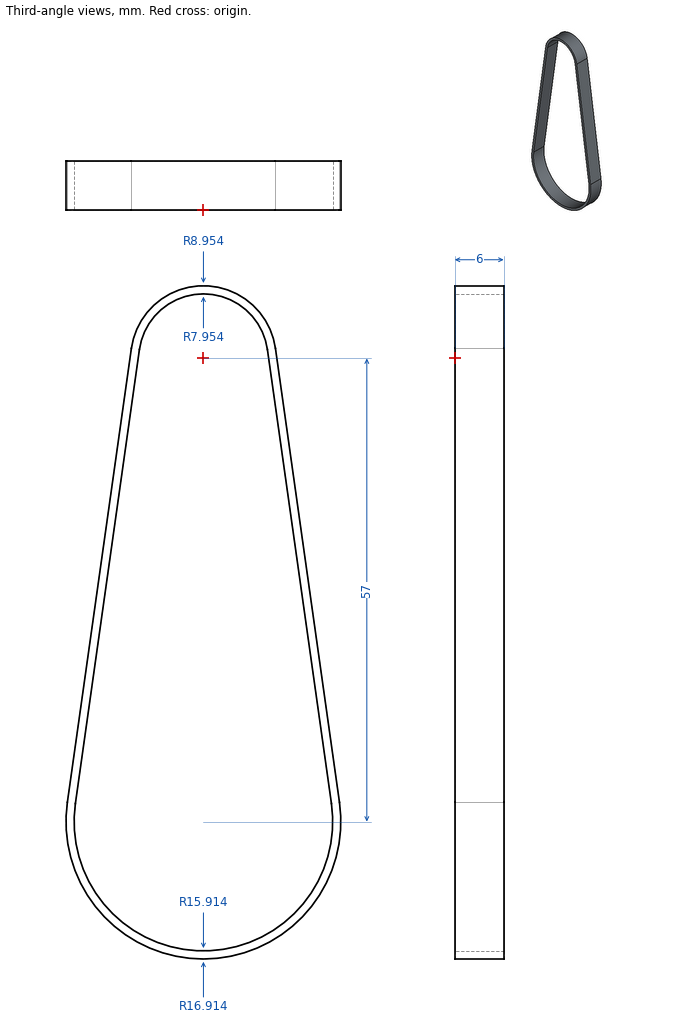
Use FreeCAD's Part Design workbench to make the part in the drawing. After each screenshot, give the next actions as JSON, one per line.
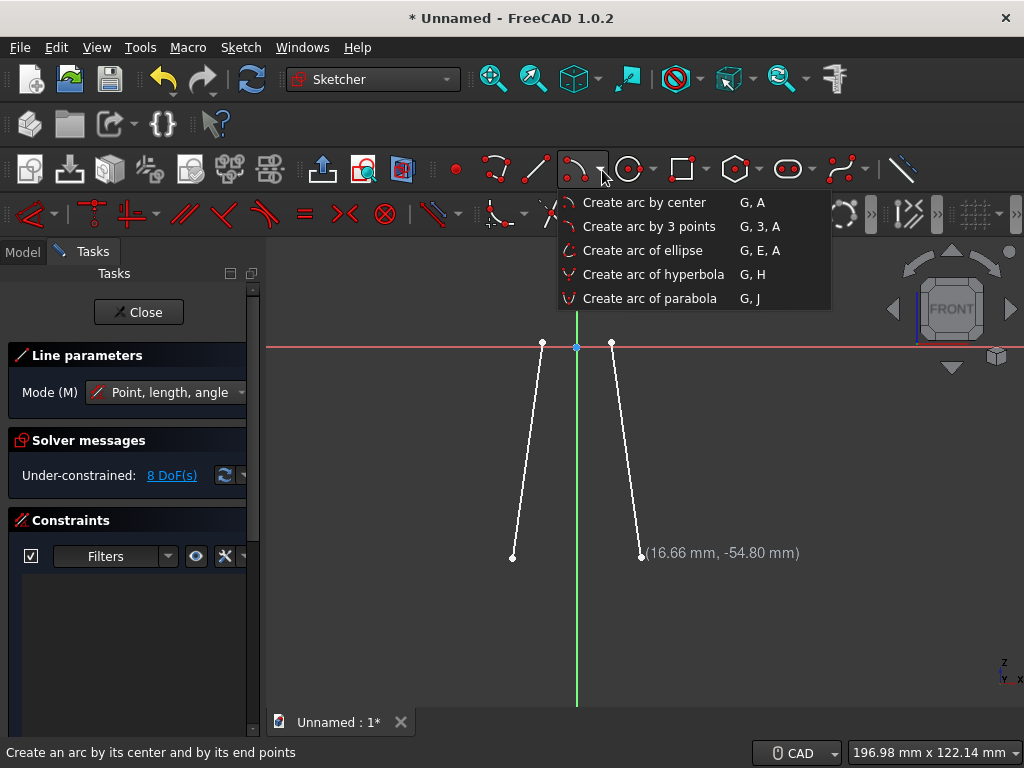
{"action": "left_click", "coordinate": [694, 226]}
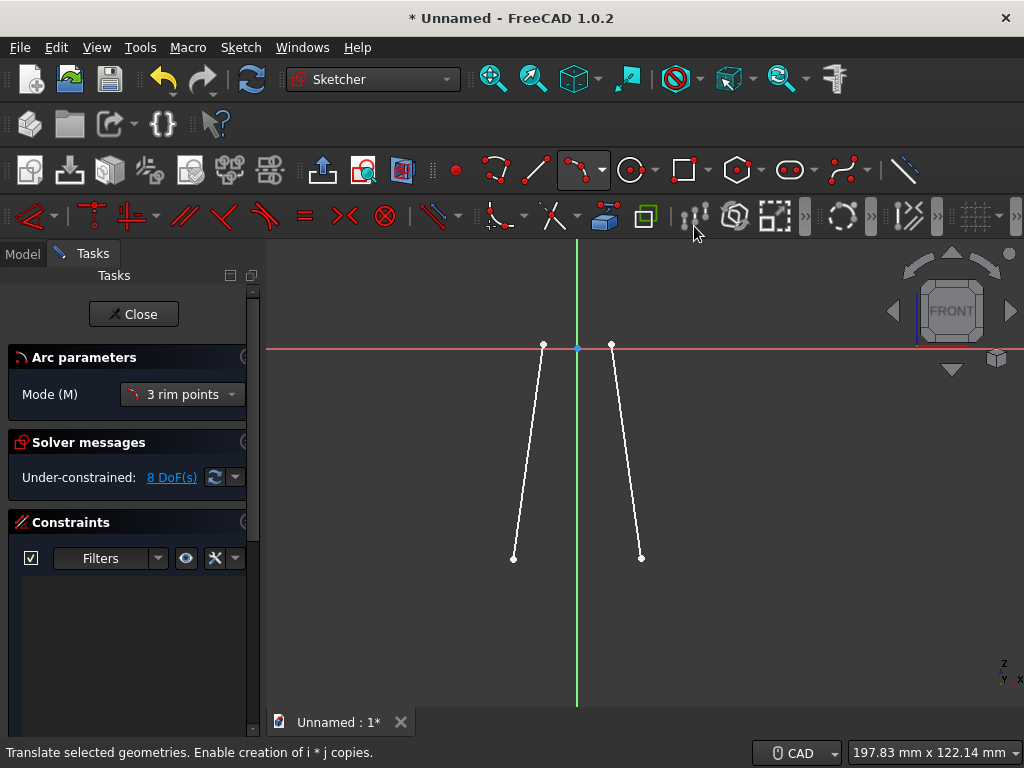
{"action": "scroll", "coordinate": [543, 344], "scroll_direction": "up", "scroll_amount": 6}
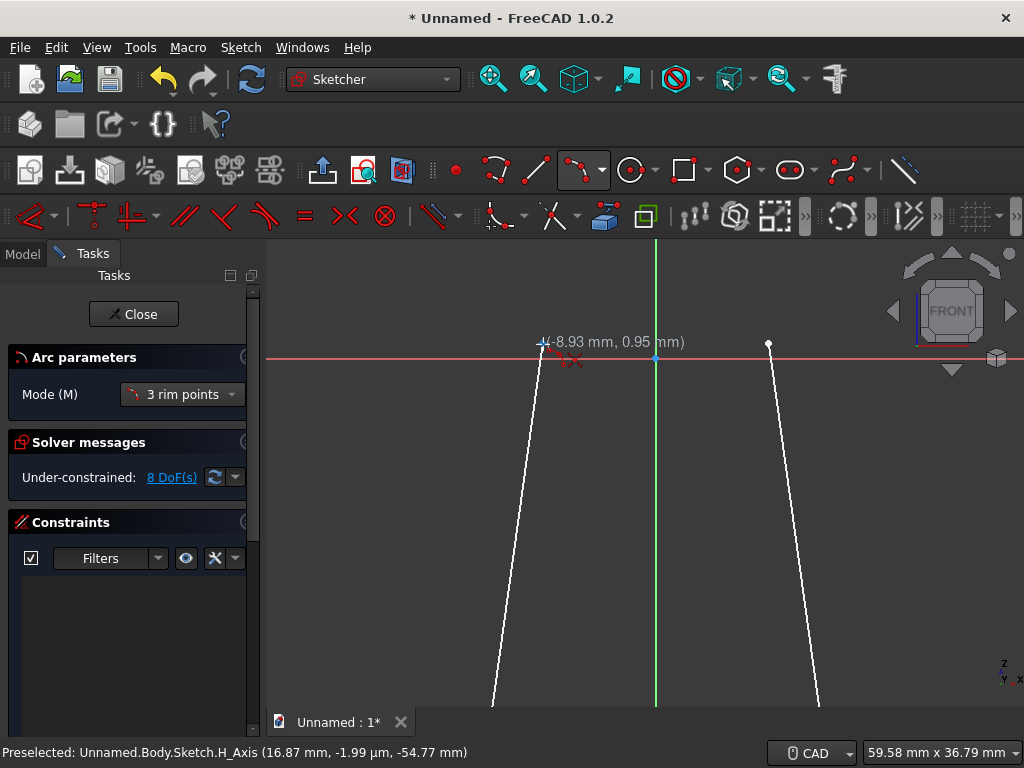
{"action": "left_click", "coordinate": [543, 344]}
{"action": "left_click", "coordinate": [769, 344]}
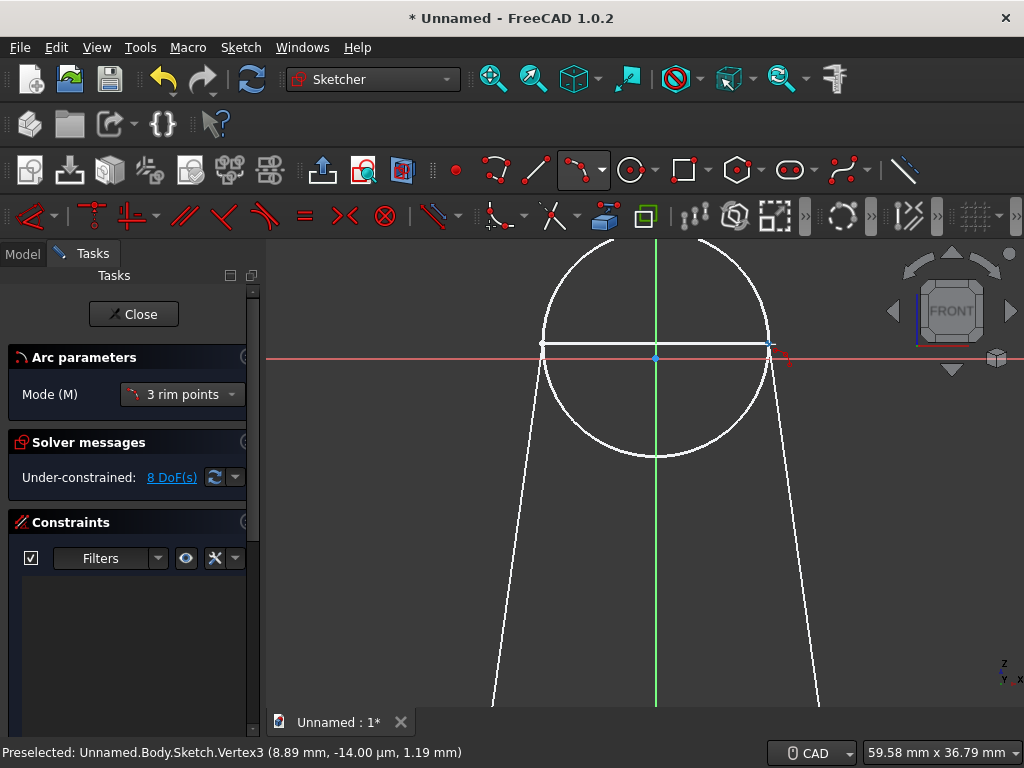
{"action": "scroll", "coordinate": [542, 344], "scroll_direction": "down", "scroll_amount": 6}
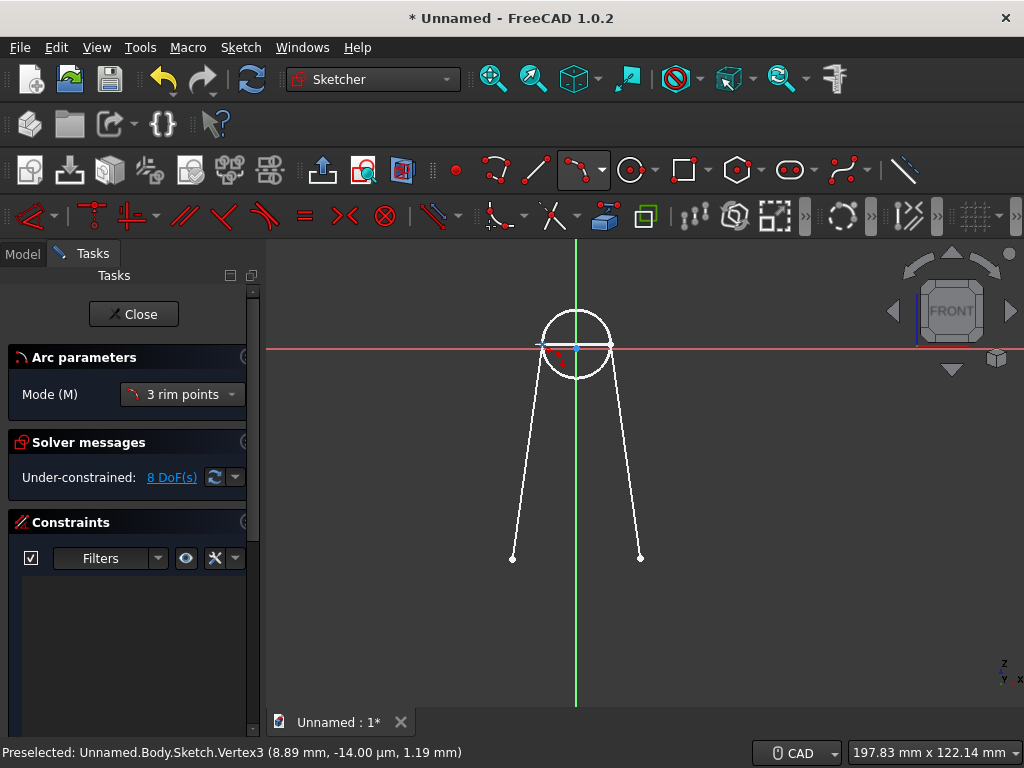
{"action": "left_click", "coordinate": [595, 320]}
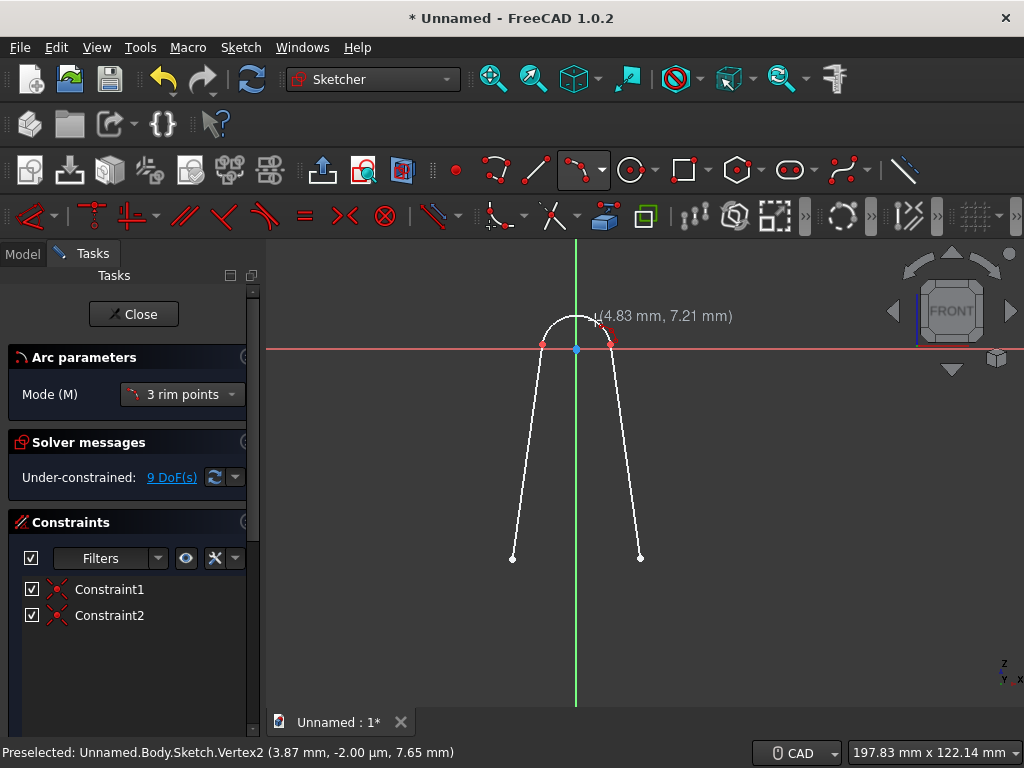
{"action": "left_click", "coordinate": [640, 559]}
{"action": "left_click", "coordinate": [513, 559]}
{"action": "left_click", "coordinate": [555, 628]}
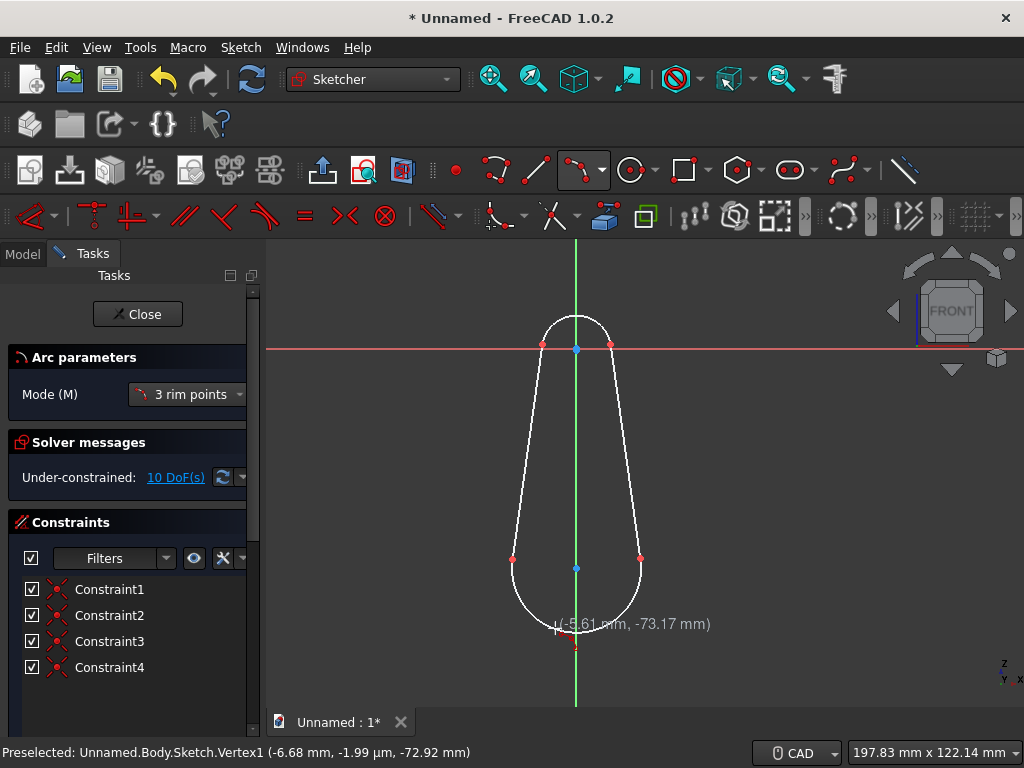
{"action": "left_click", "coordinate": [536, 170]}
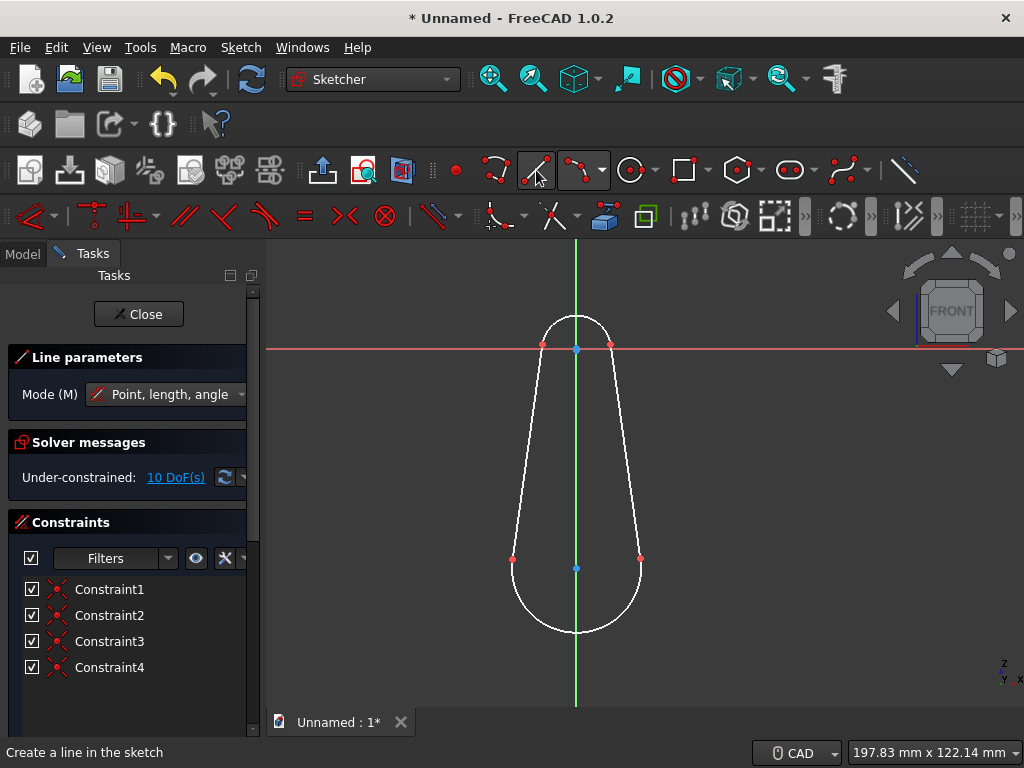
{"action": "scroll", "coordinate": [546, 344], "scroll_direction": "up", "scroll_amount": 8}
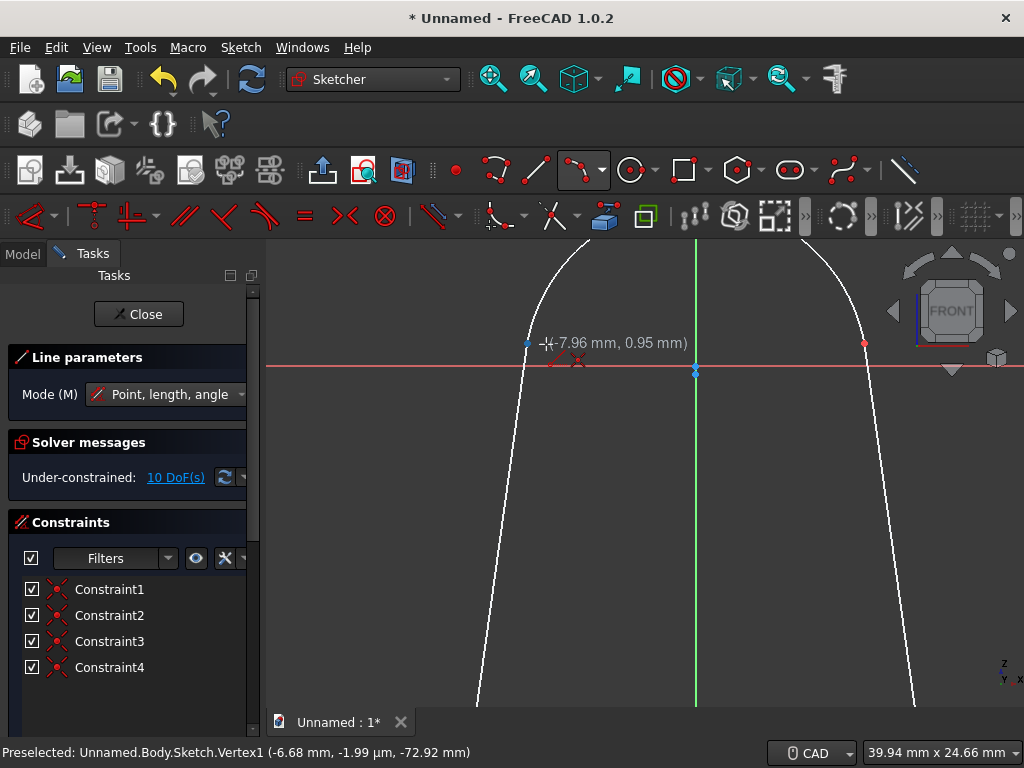
{"action": "left_click", "coordinate": [546, 345]}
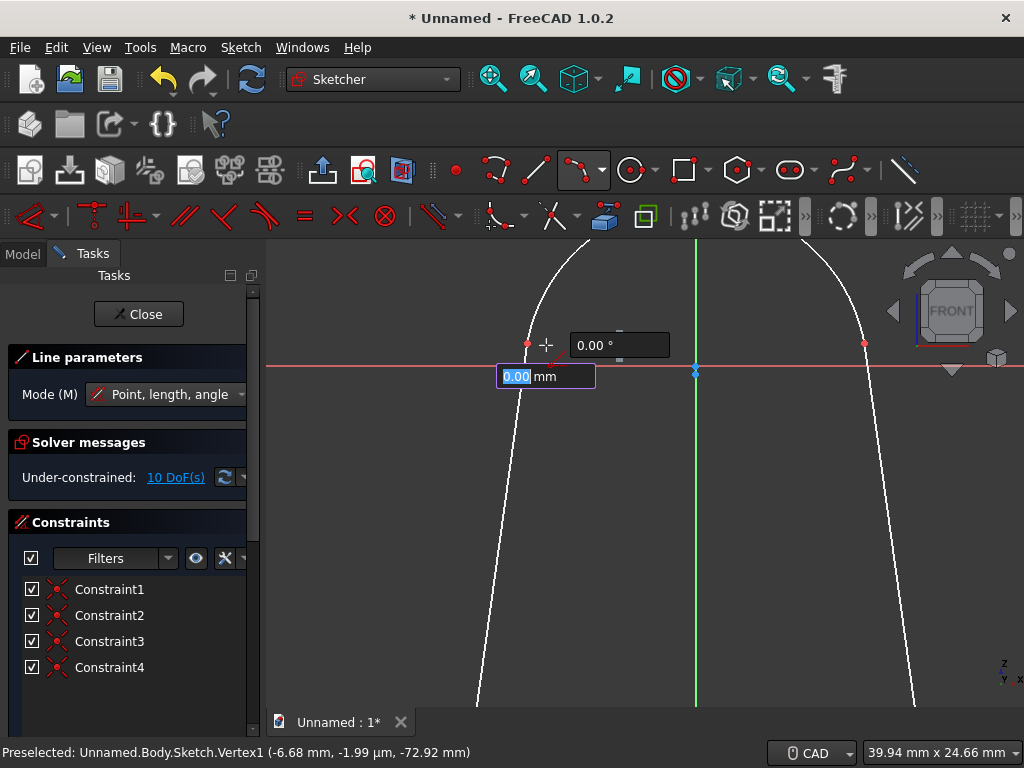
{"action": "scroll", "coordinate": [546, 344], "scroll_direction": "down", "scroll_amount": 8}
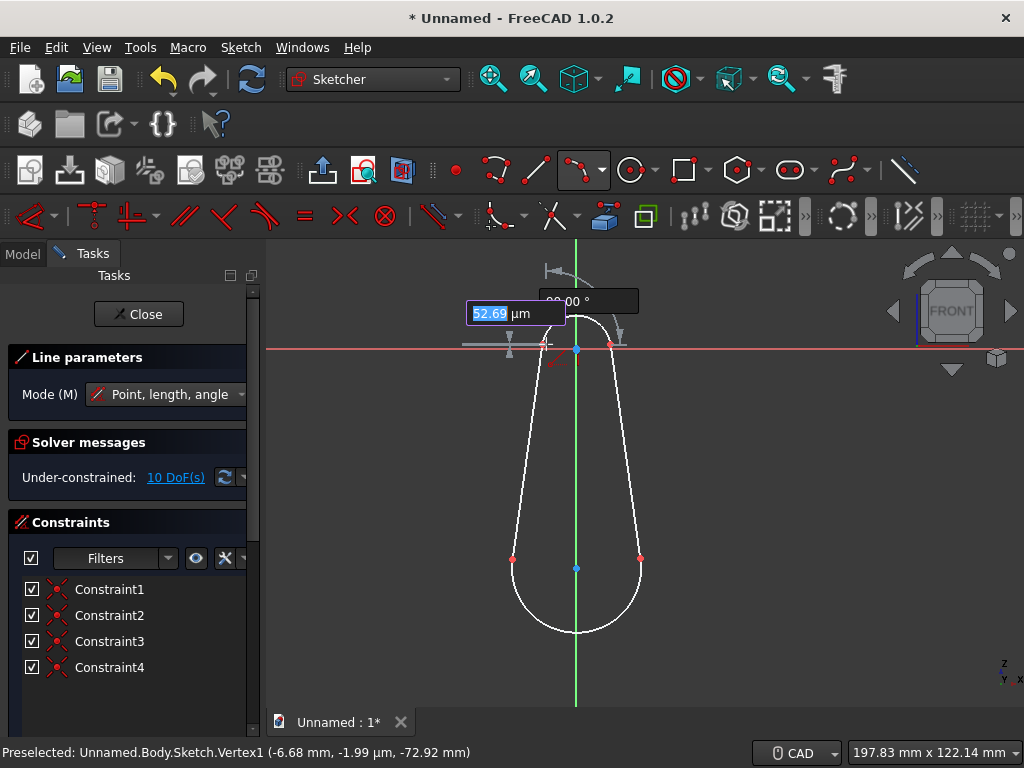
{"action": "scroll", "coordinate": [516, 559], "scroll_direction": "up", "scroll_amount": 8}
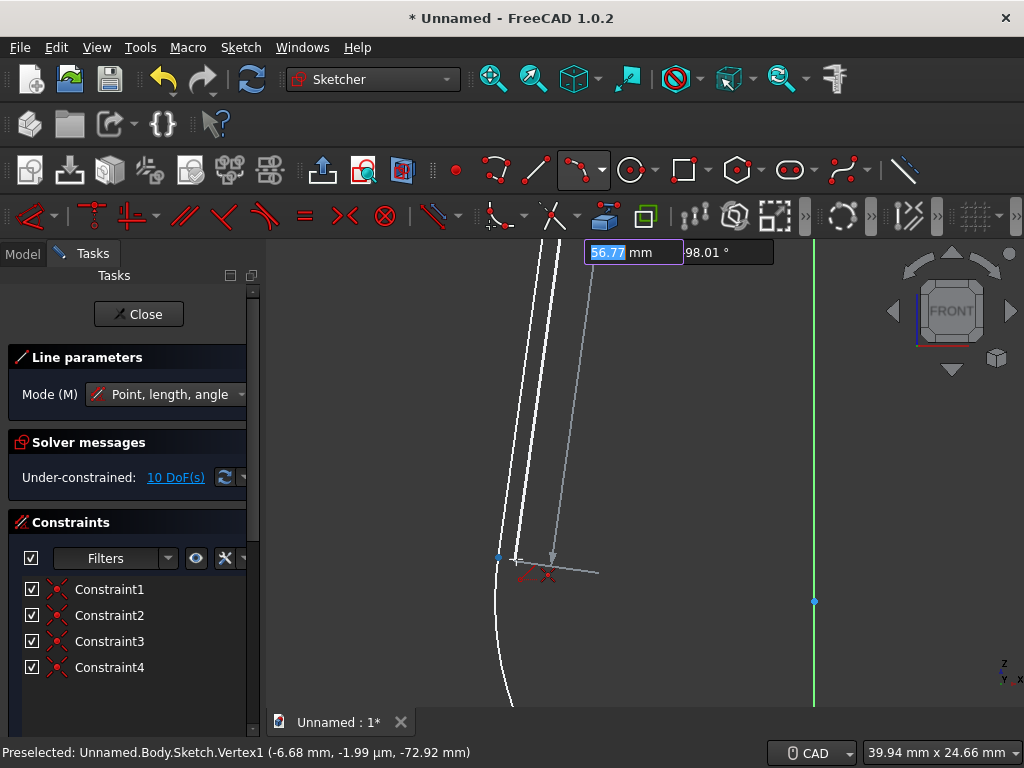
{"action": "left_click", "coordinate": [515, 554]}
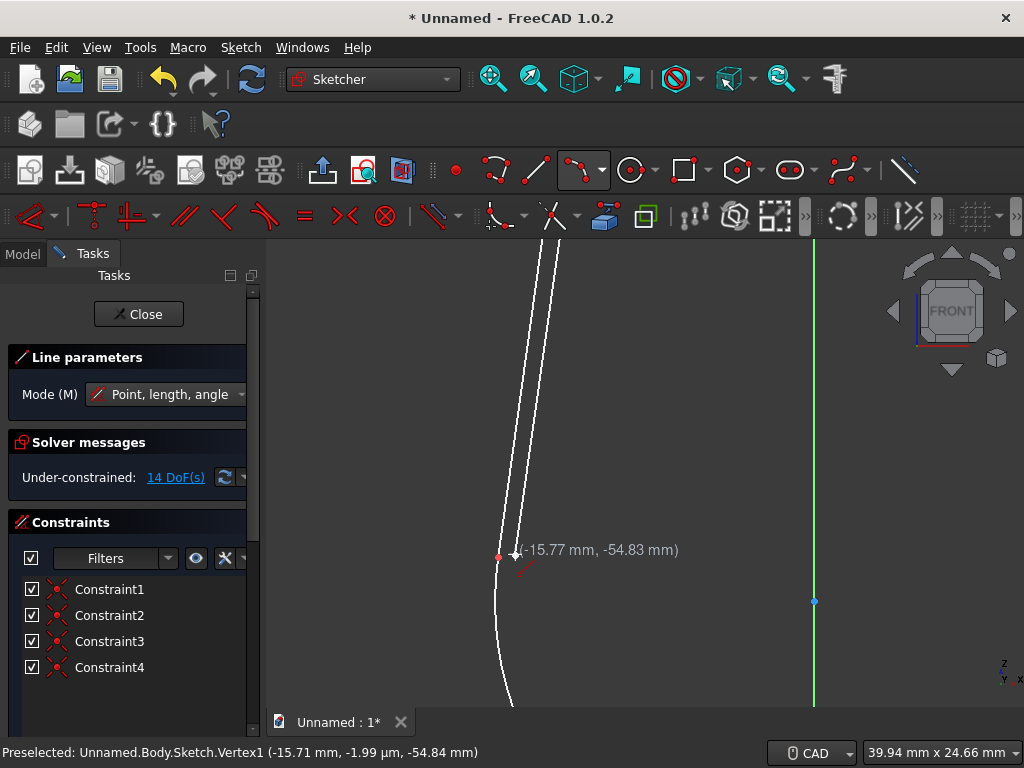
{"action": "scroll", "coordinate": [516, 560], "scroll_direction": "down", "scroll_amount": 8}